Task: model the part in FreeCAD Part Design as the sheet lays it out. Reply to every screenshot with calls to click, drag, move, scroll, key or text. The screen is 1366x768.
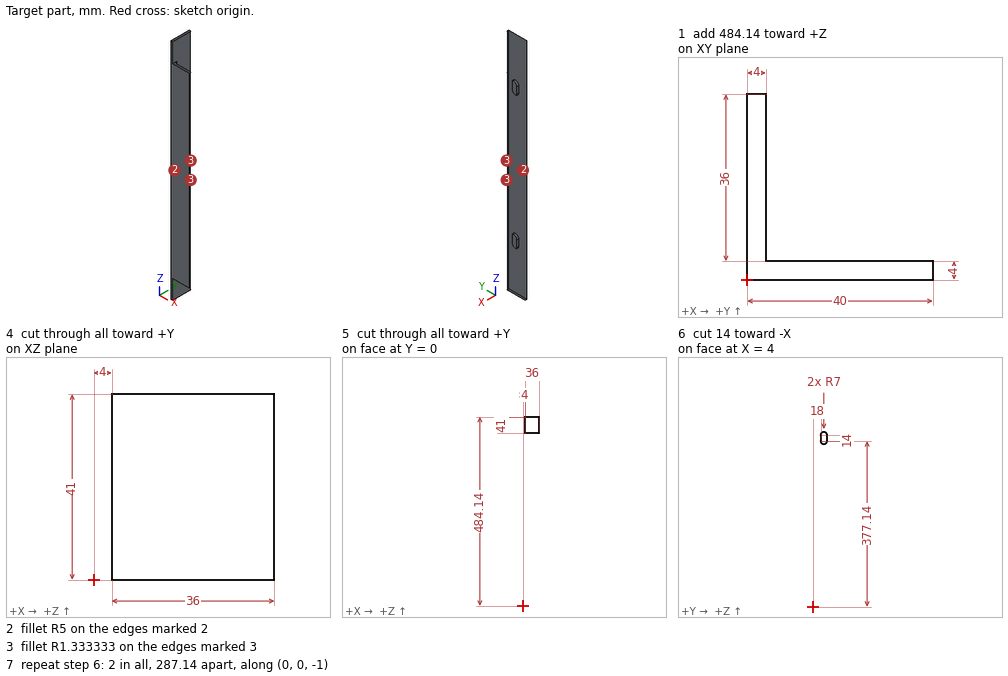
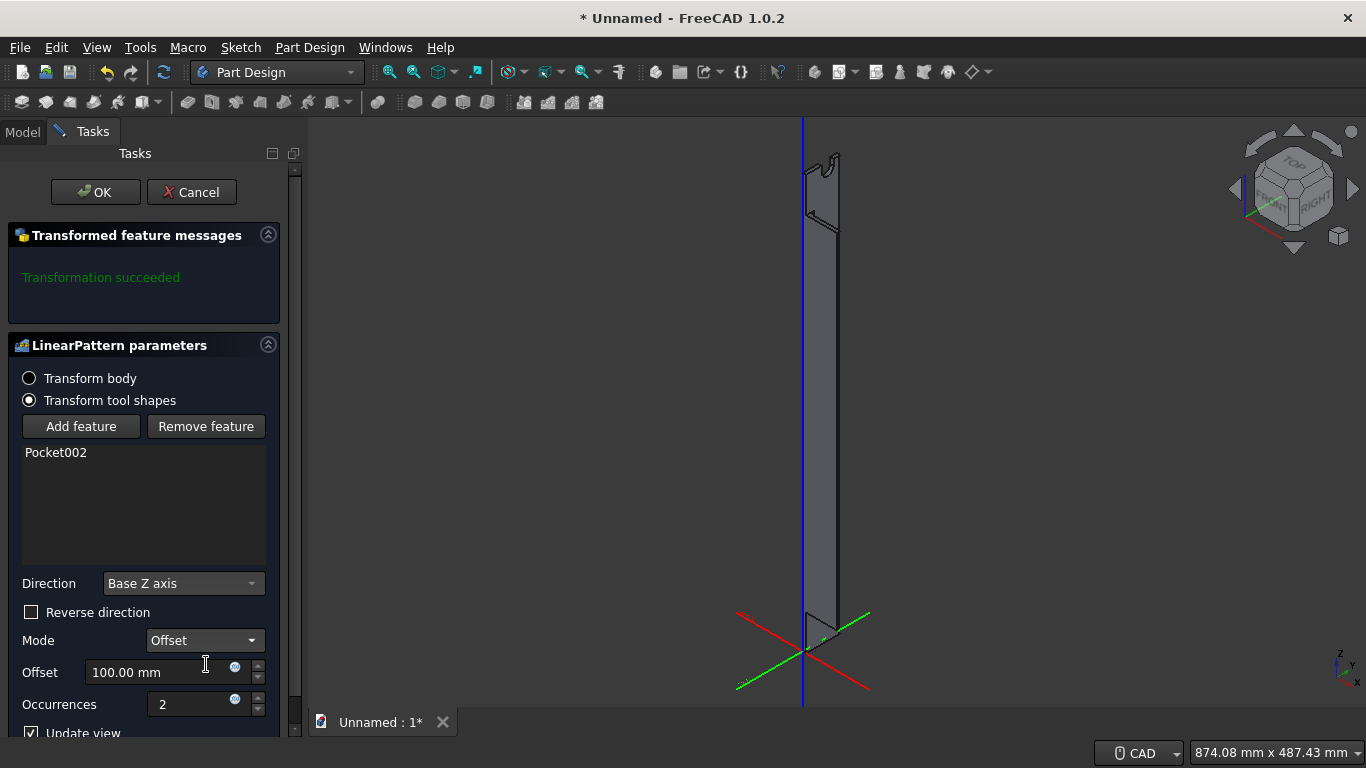
triple_click(168, 672)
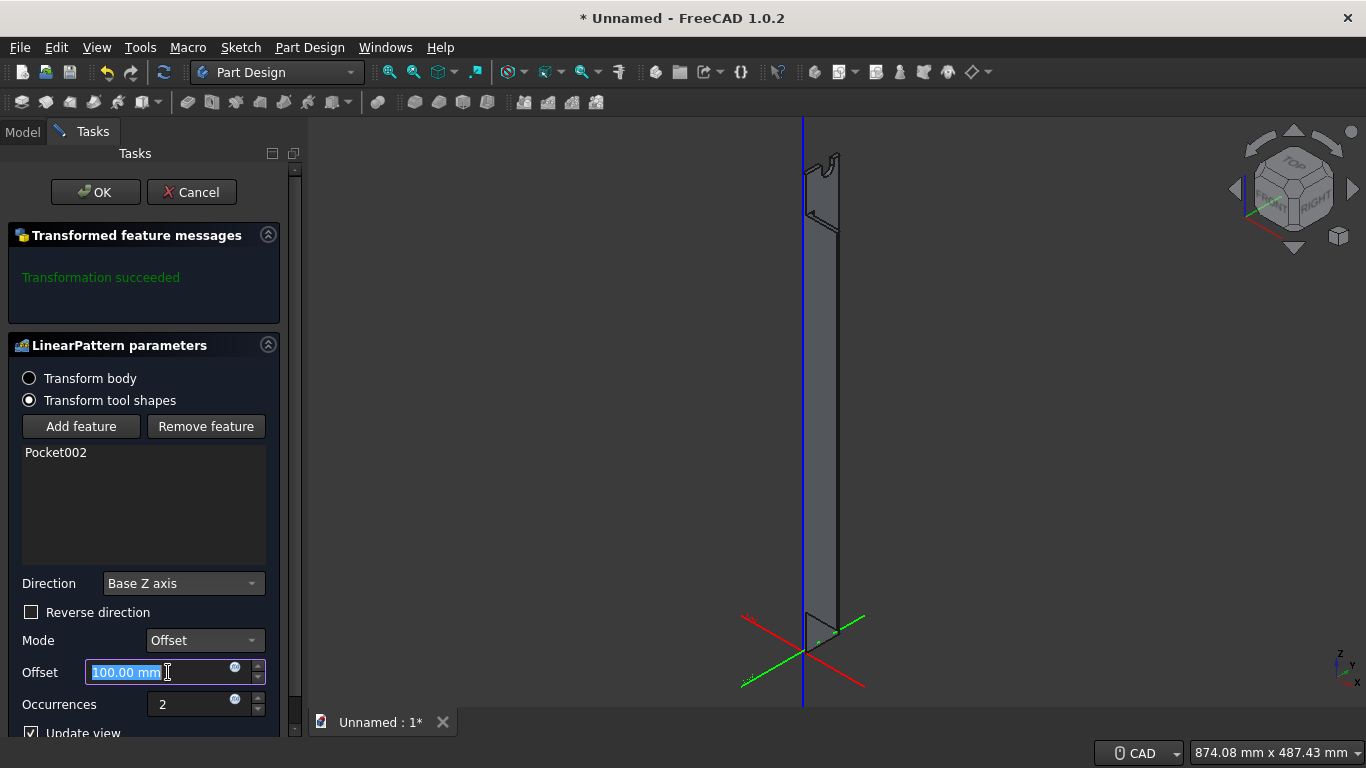
text(287.14)
key(Tab)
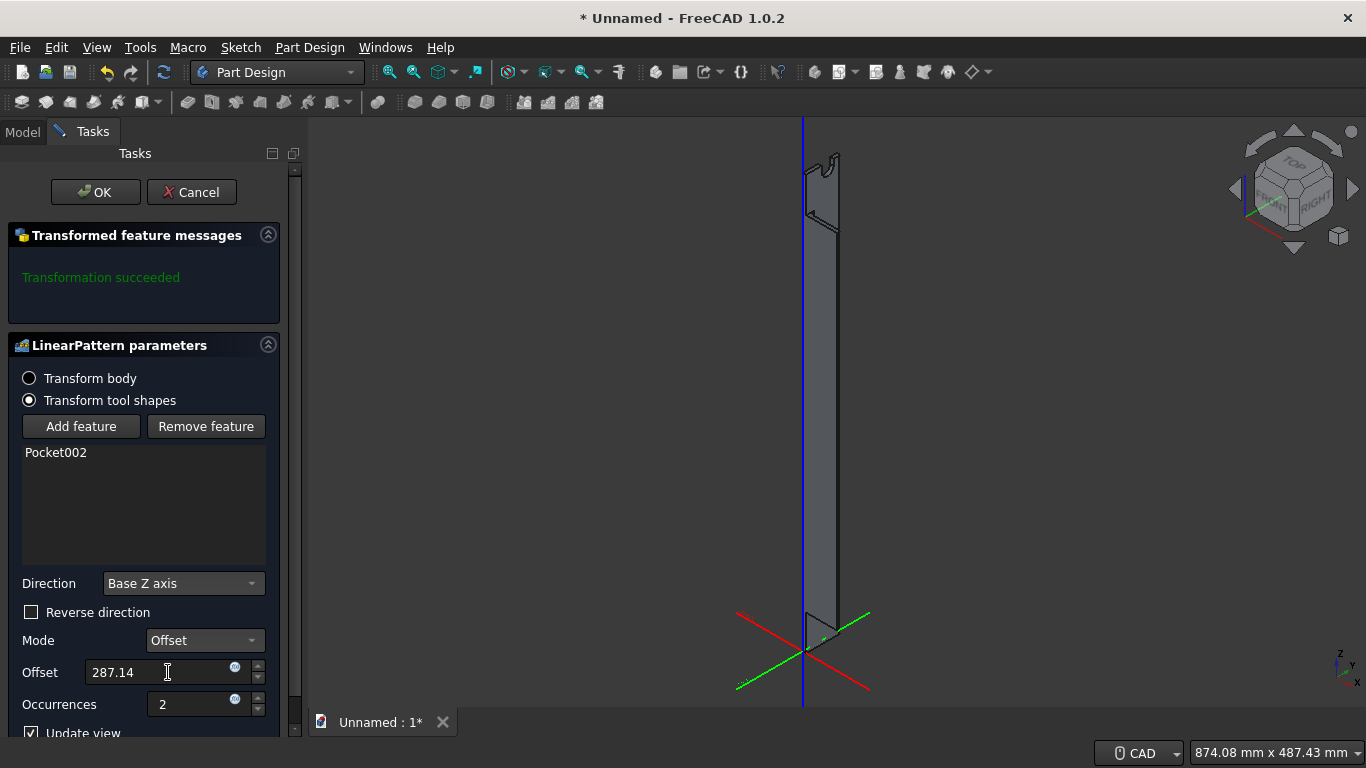
triple_click(198, 704)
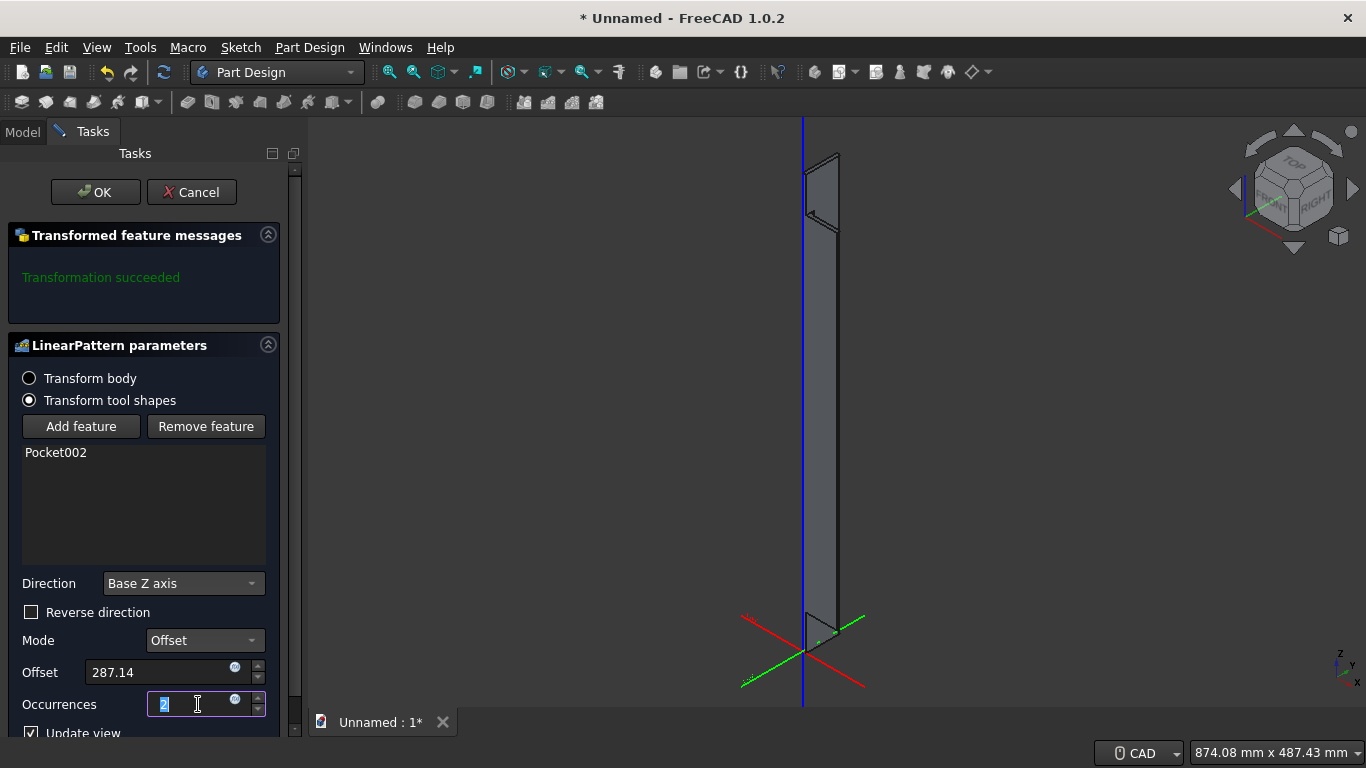
text(2)
key(Tab)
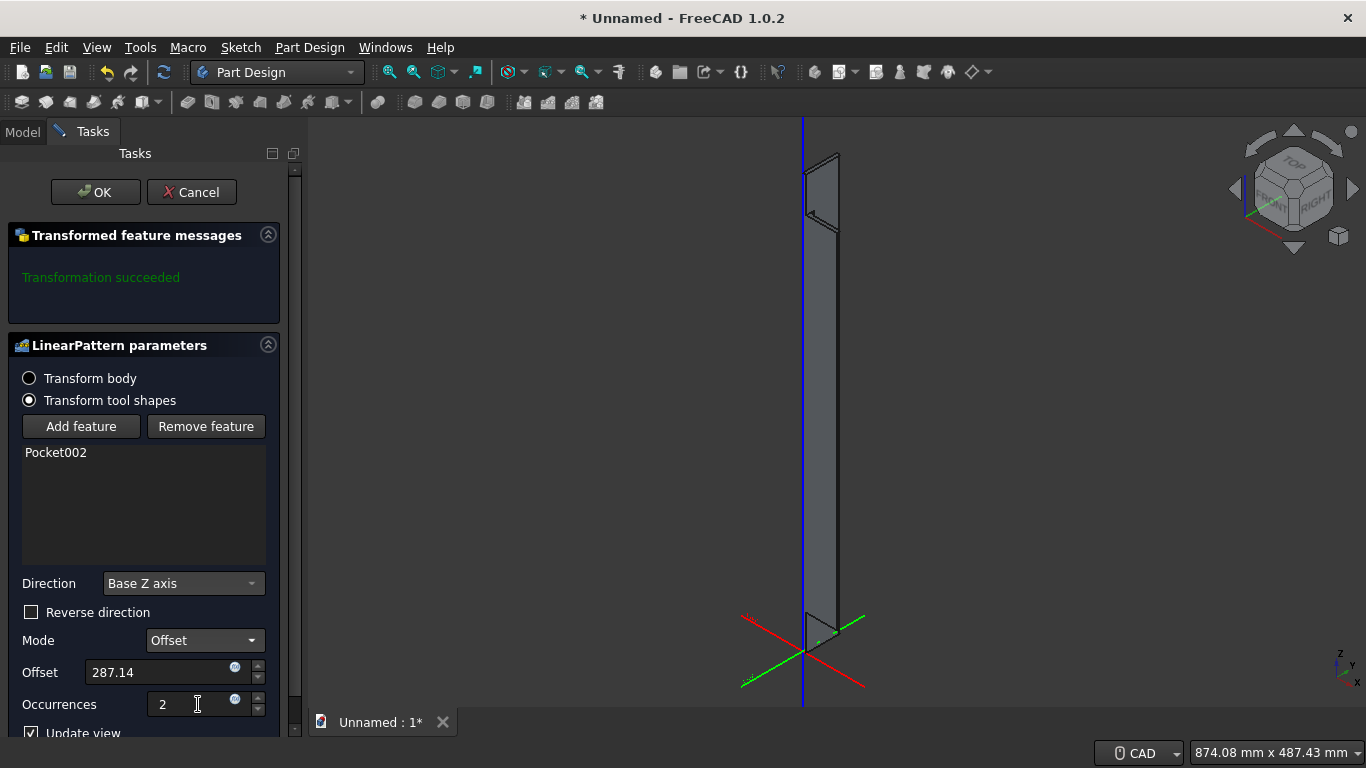
click(30, 612)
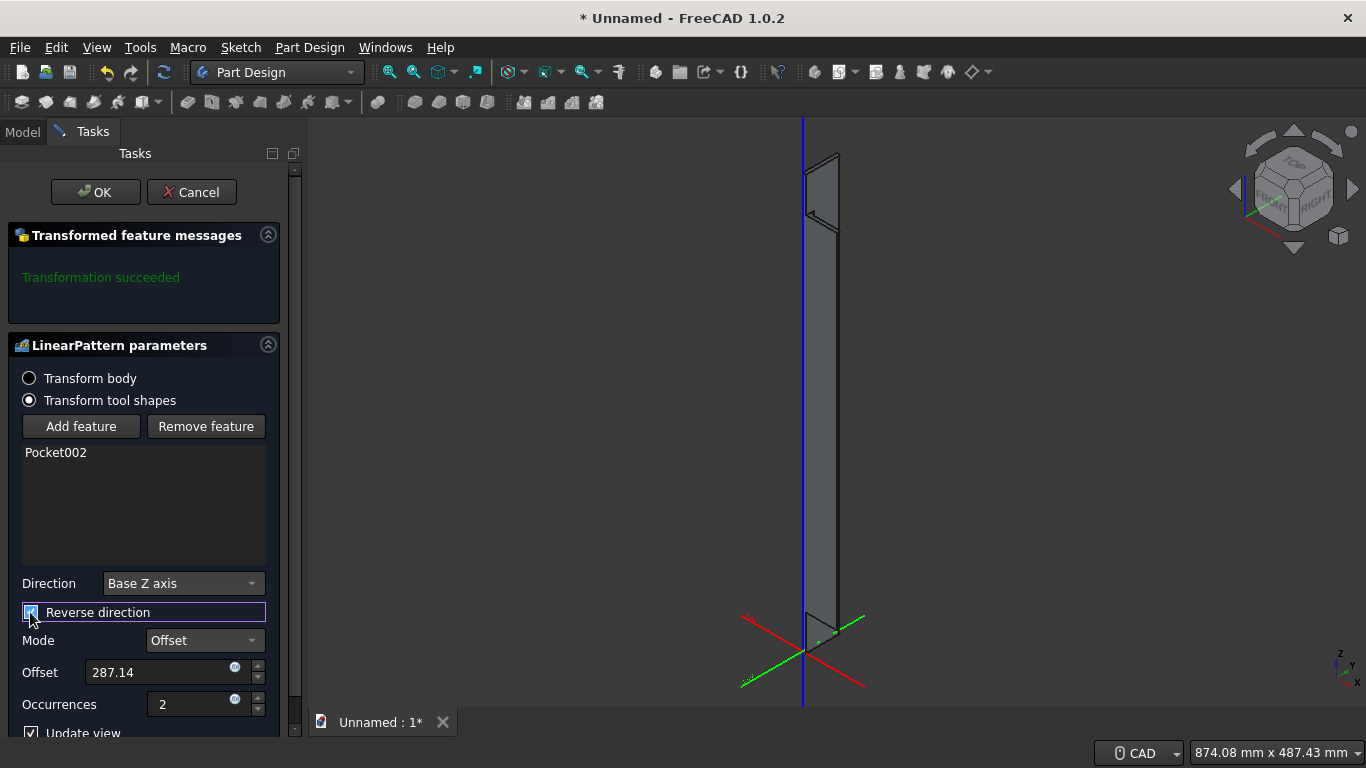
click(96, 192)